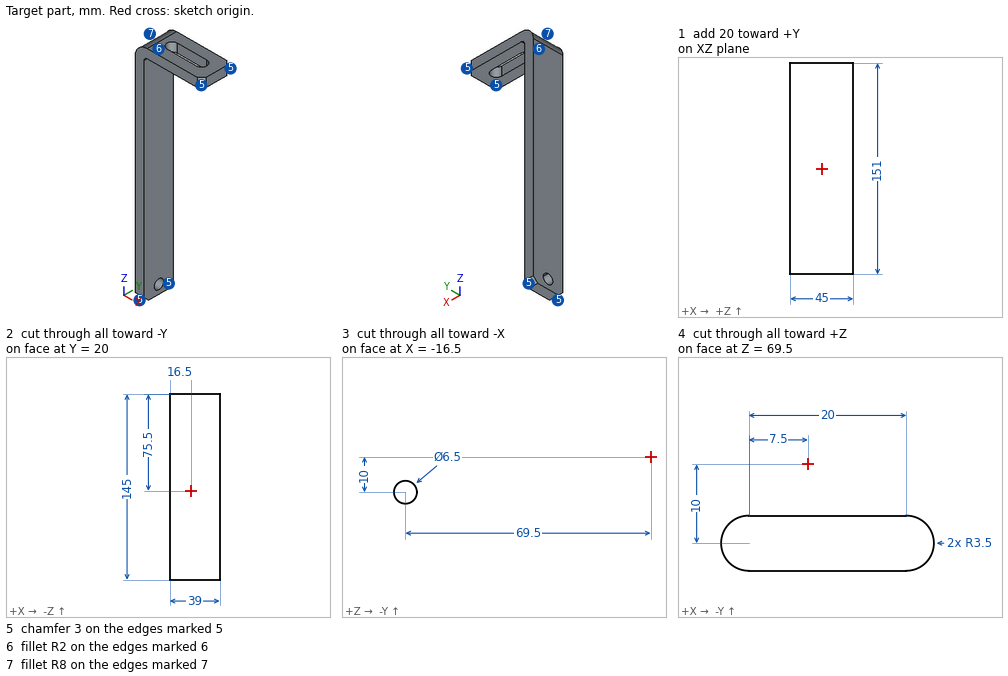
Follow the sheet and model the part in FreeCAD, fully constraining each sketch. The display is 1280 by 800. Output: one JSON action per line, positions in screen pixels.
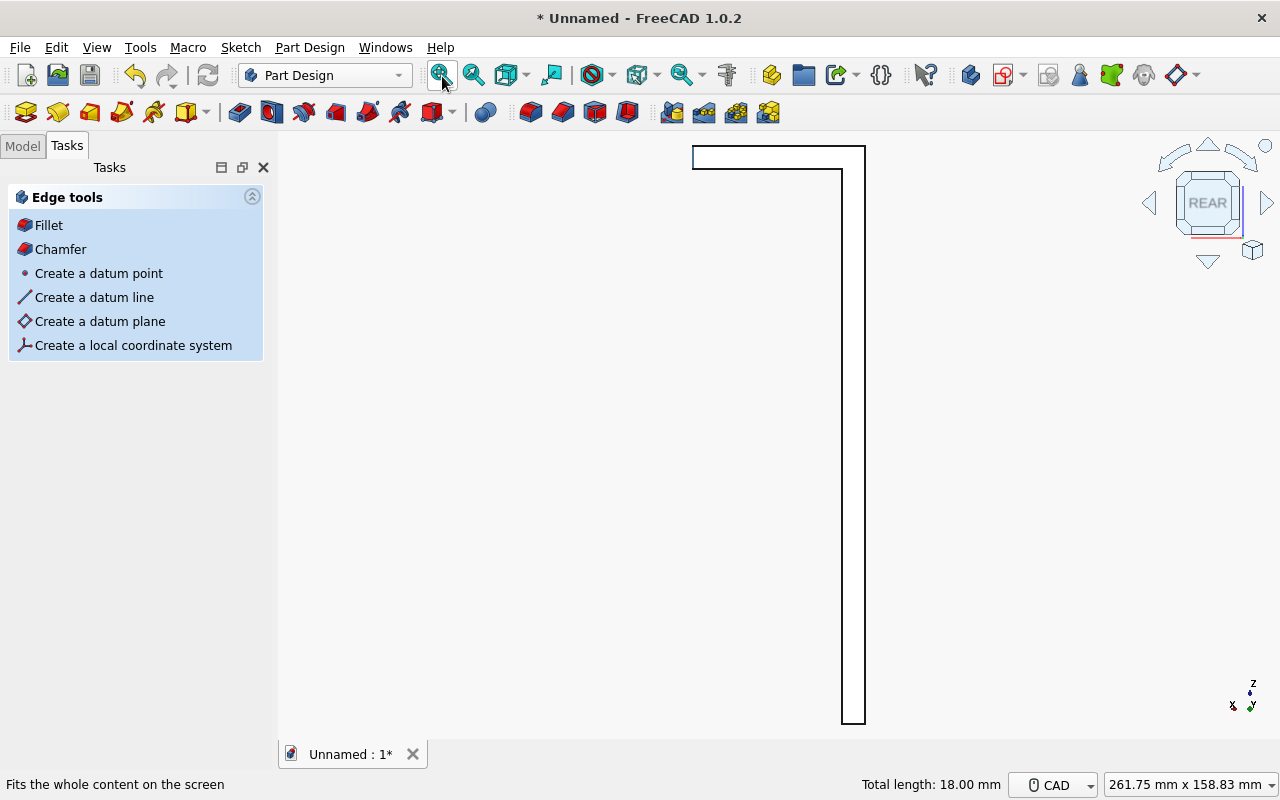
{"action": "key", "text": "6"}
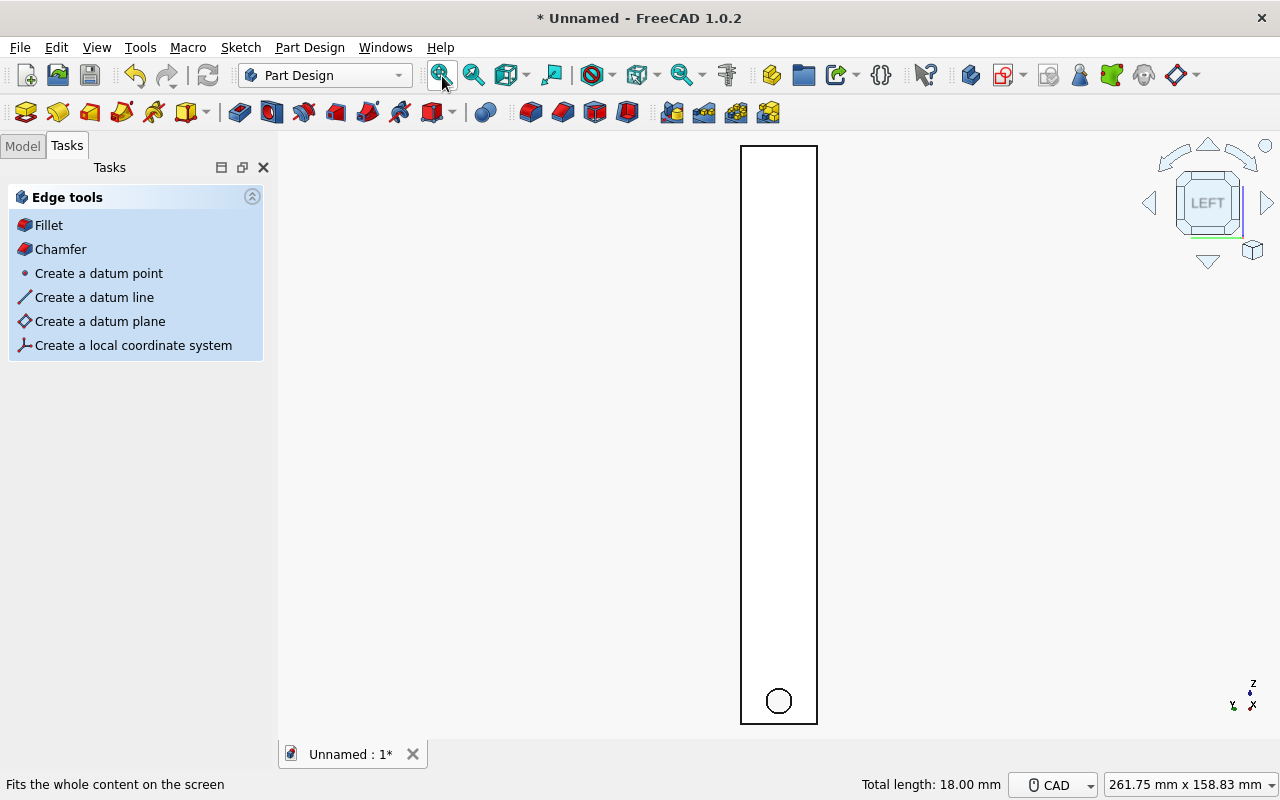
{"action": "key", "text": "v 3"}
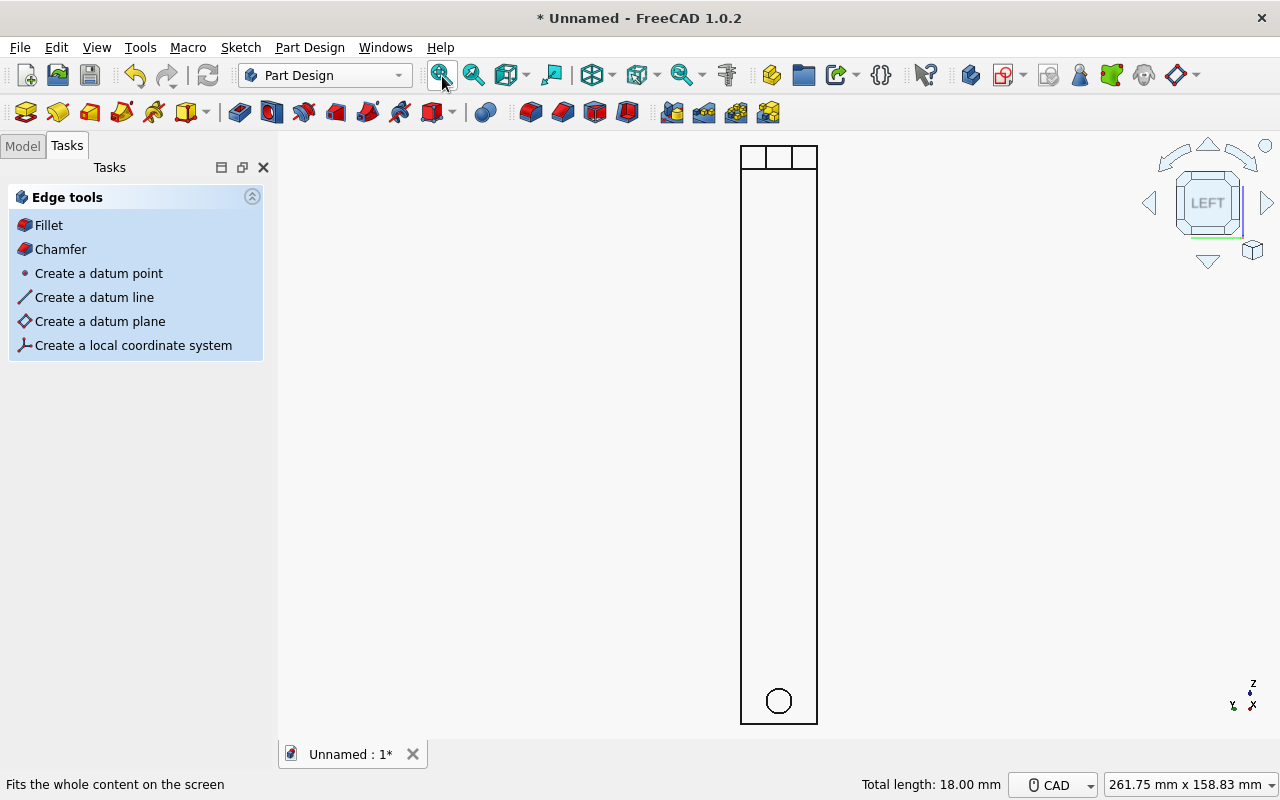
{"action": "key", "text": "0"}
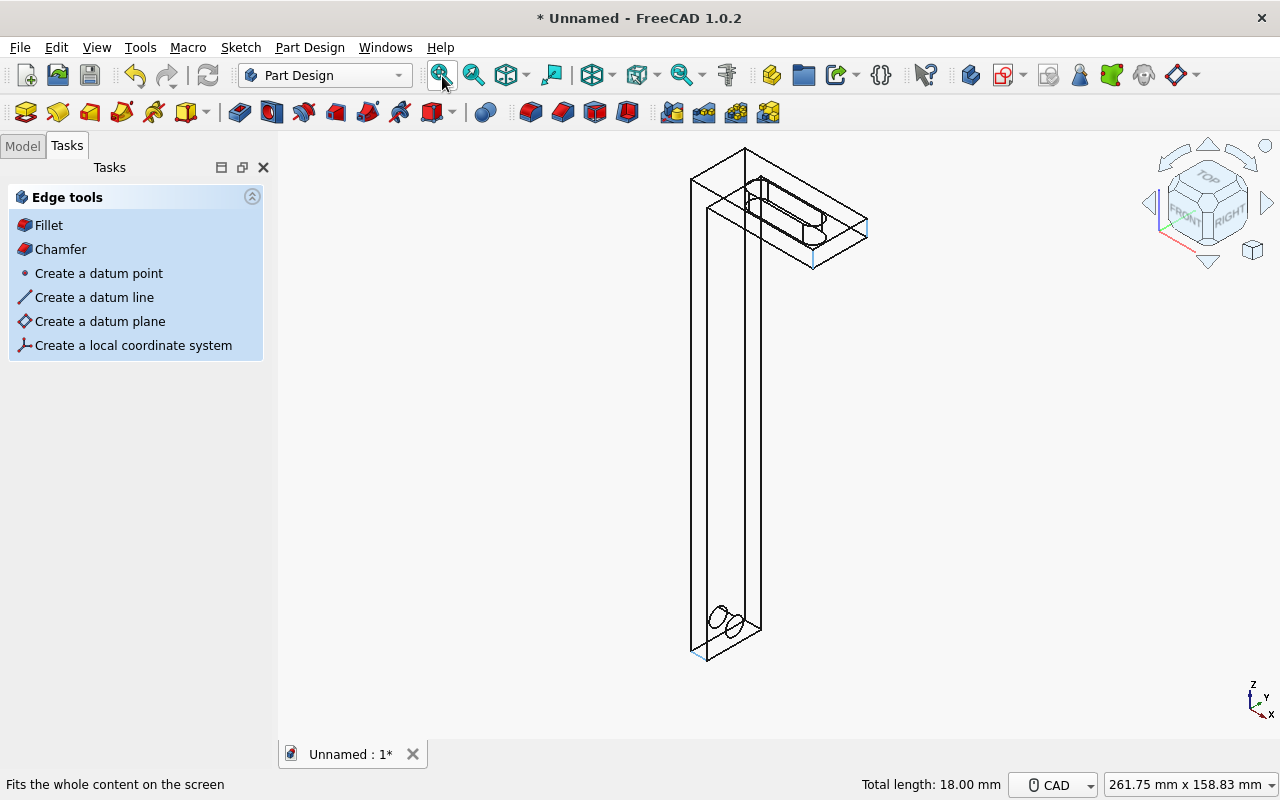
{"action": "left_click", "coordinate": [753, 624], "text": "ctrl"}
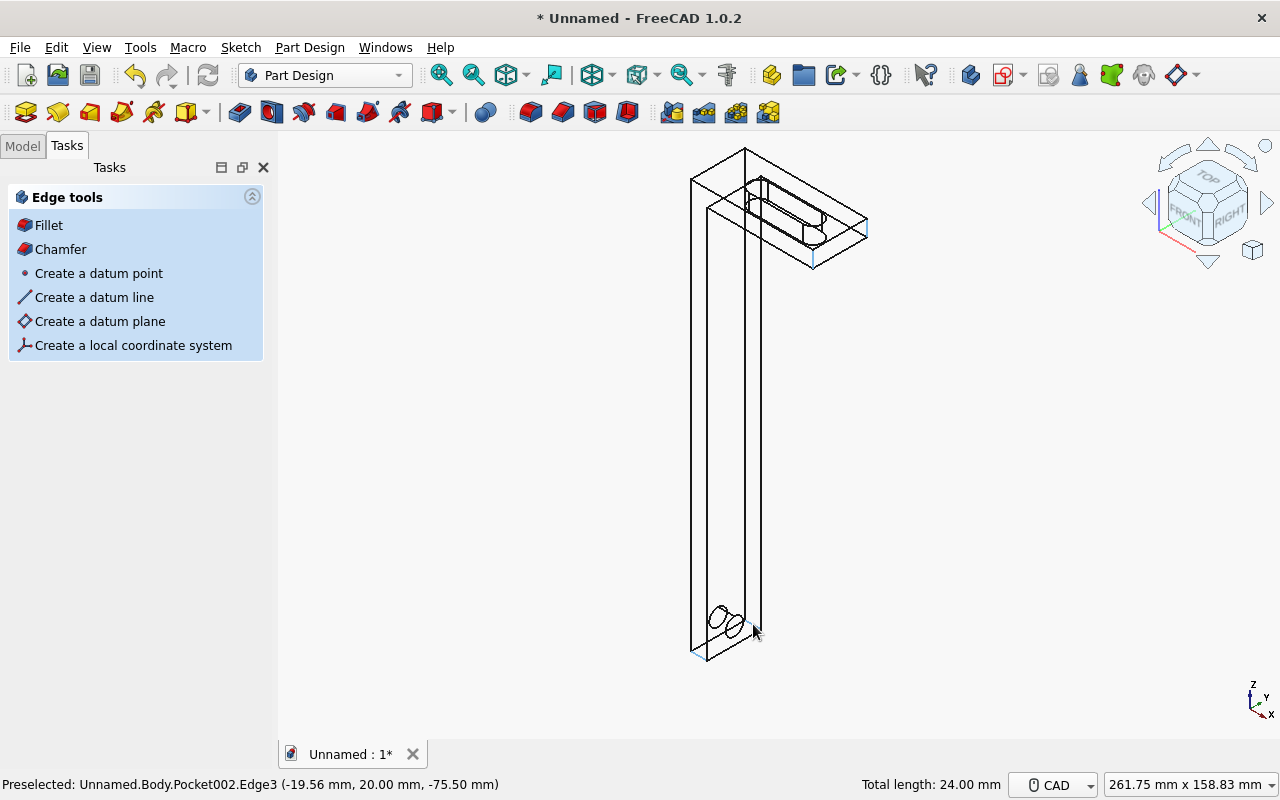
{"action": "key", "text": "v 1"}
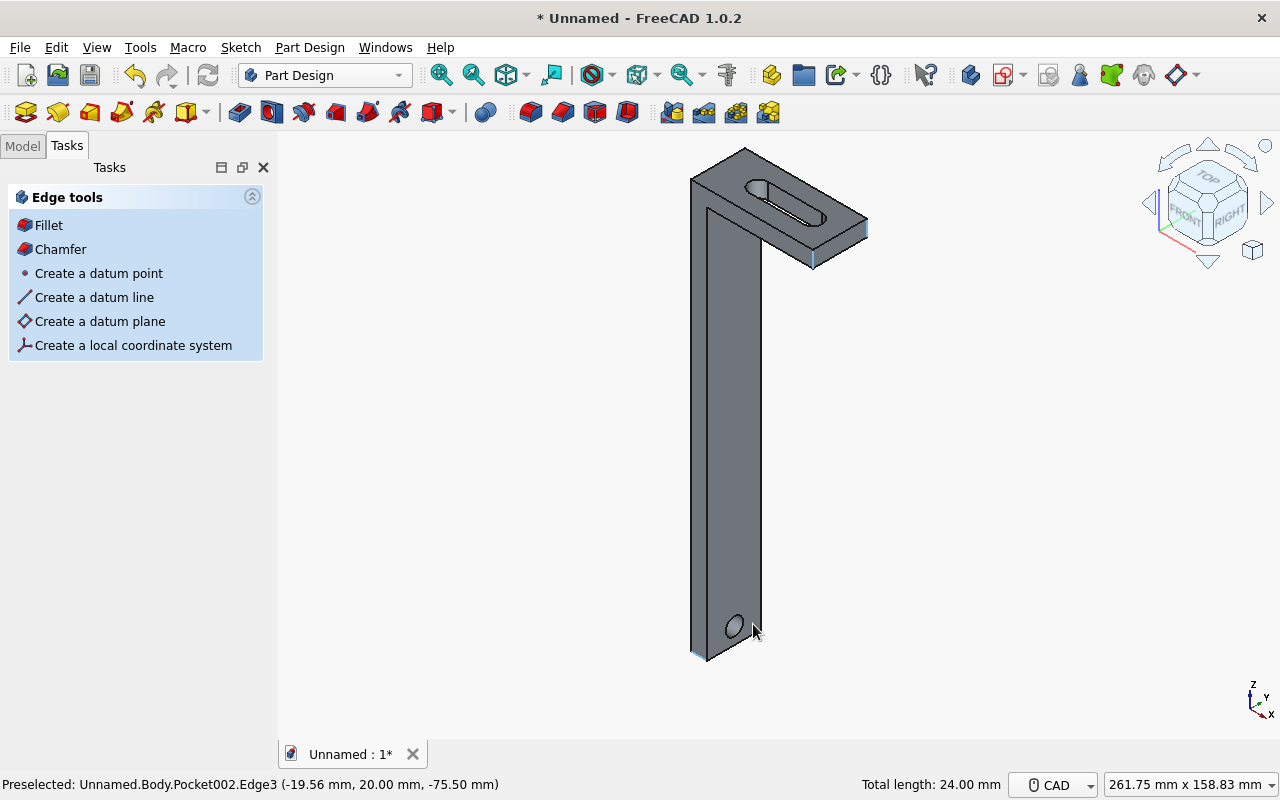
{"action": "left_click", "coordinate": [564, 112]}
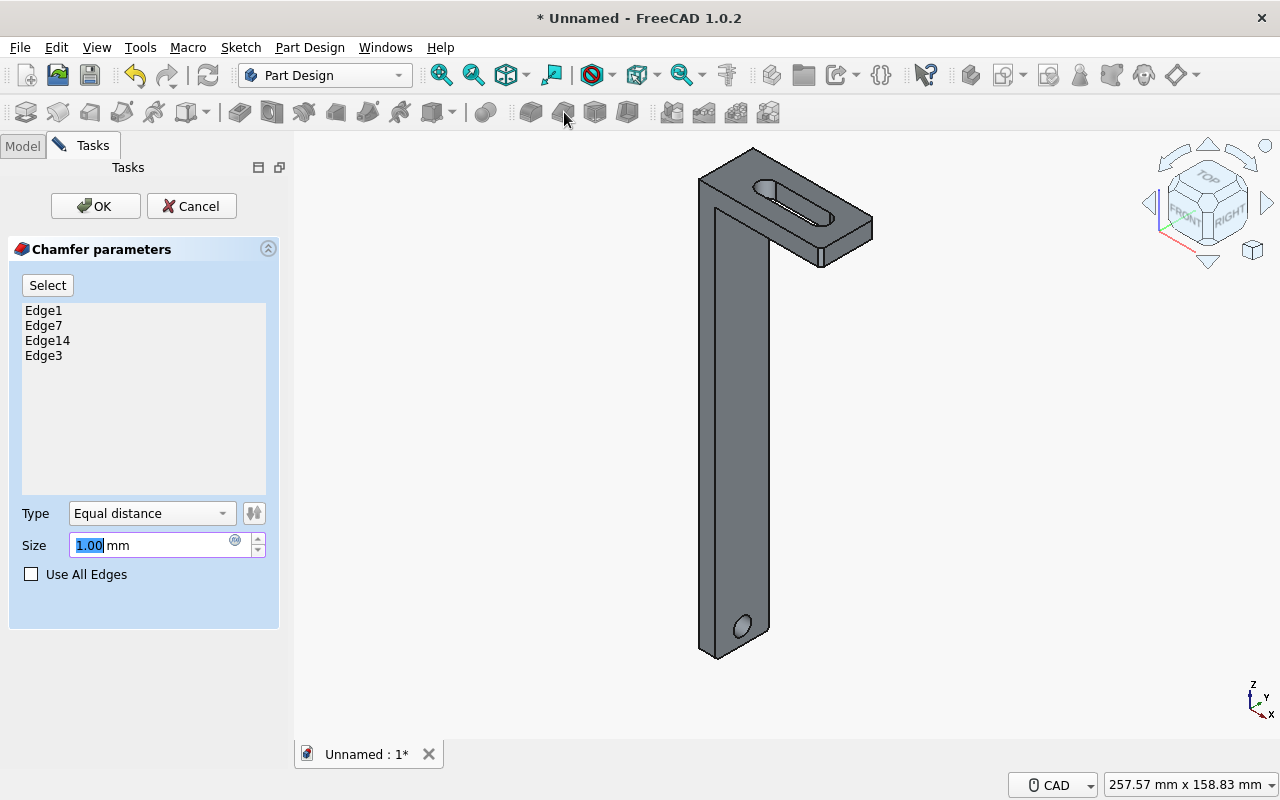
{"action": "type", "text": "3"}
{"action": "key", "text": "Tab"}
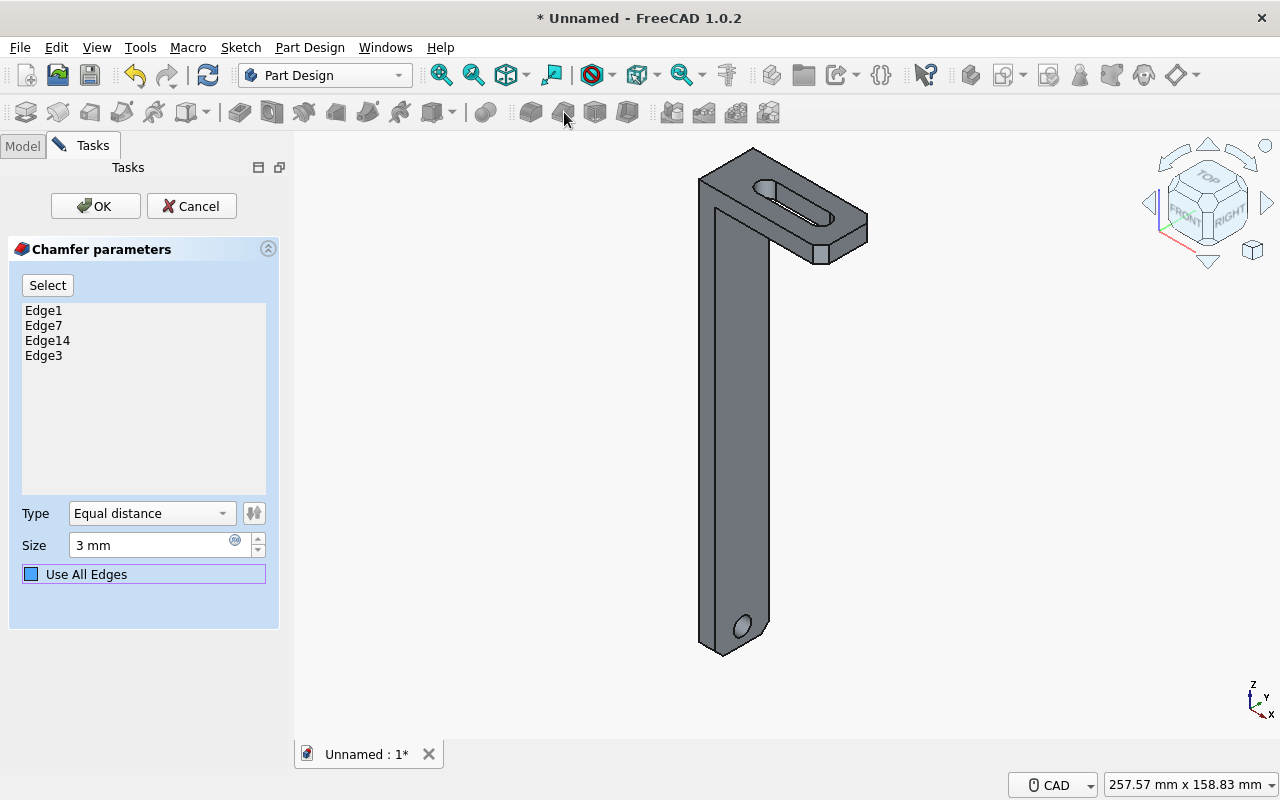
{"action": "left_click", "coordinate": [96, 206]}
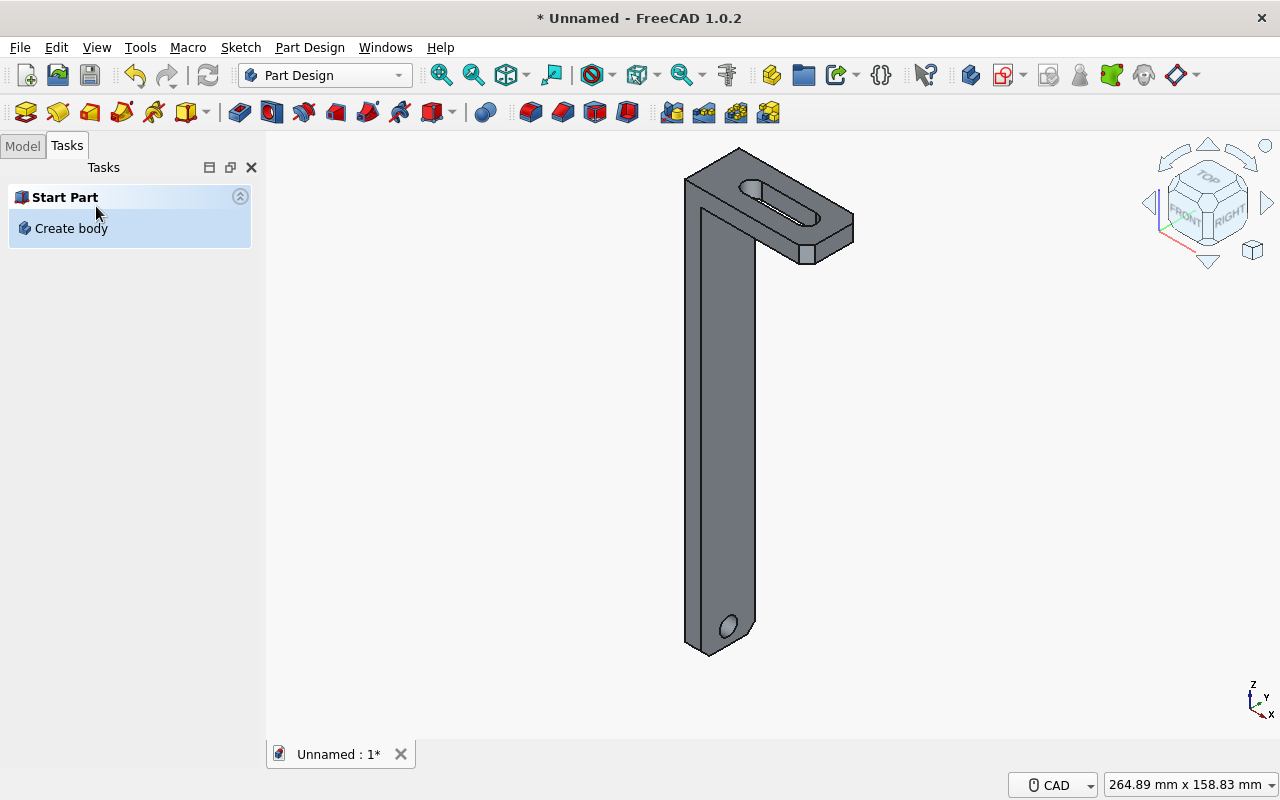
{"action": "key", "text": "2"}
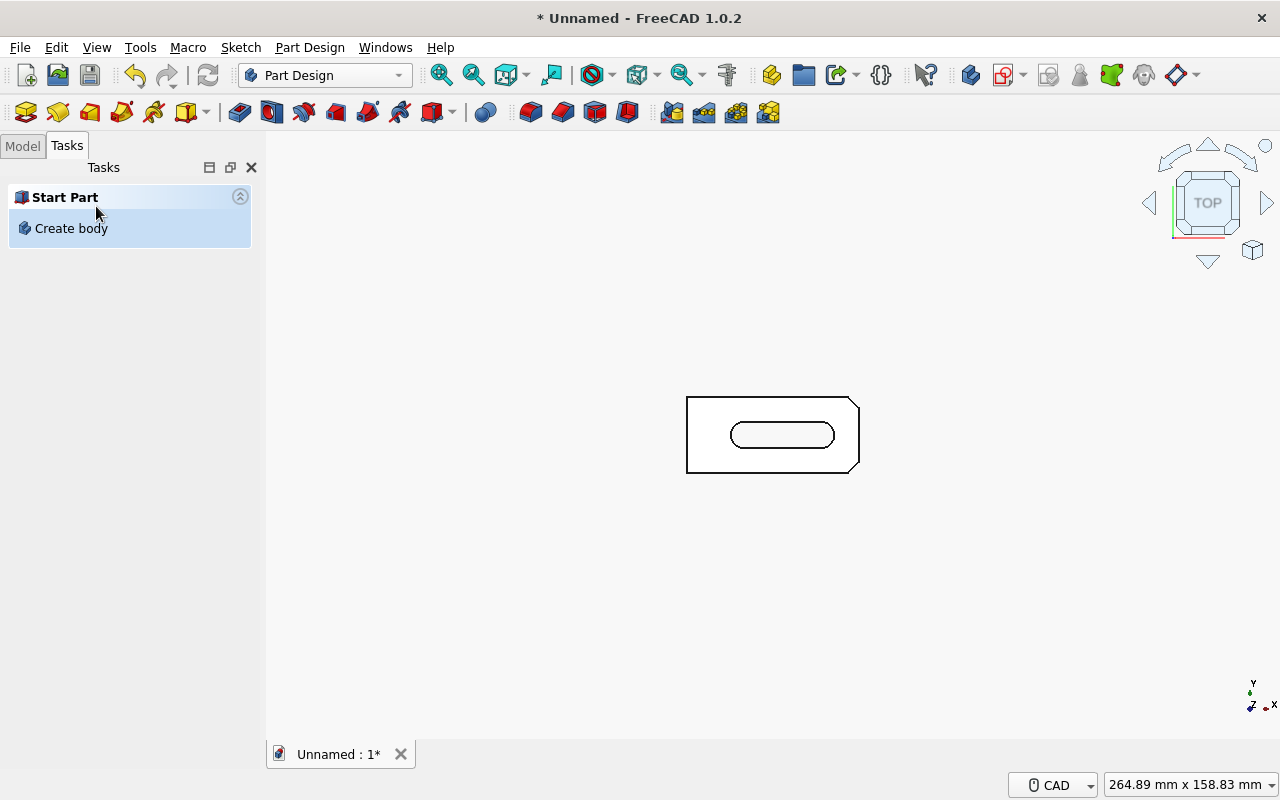
{"action": "left_click", "coordinate": [442, 76]}